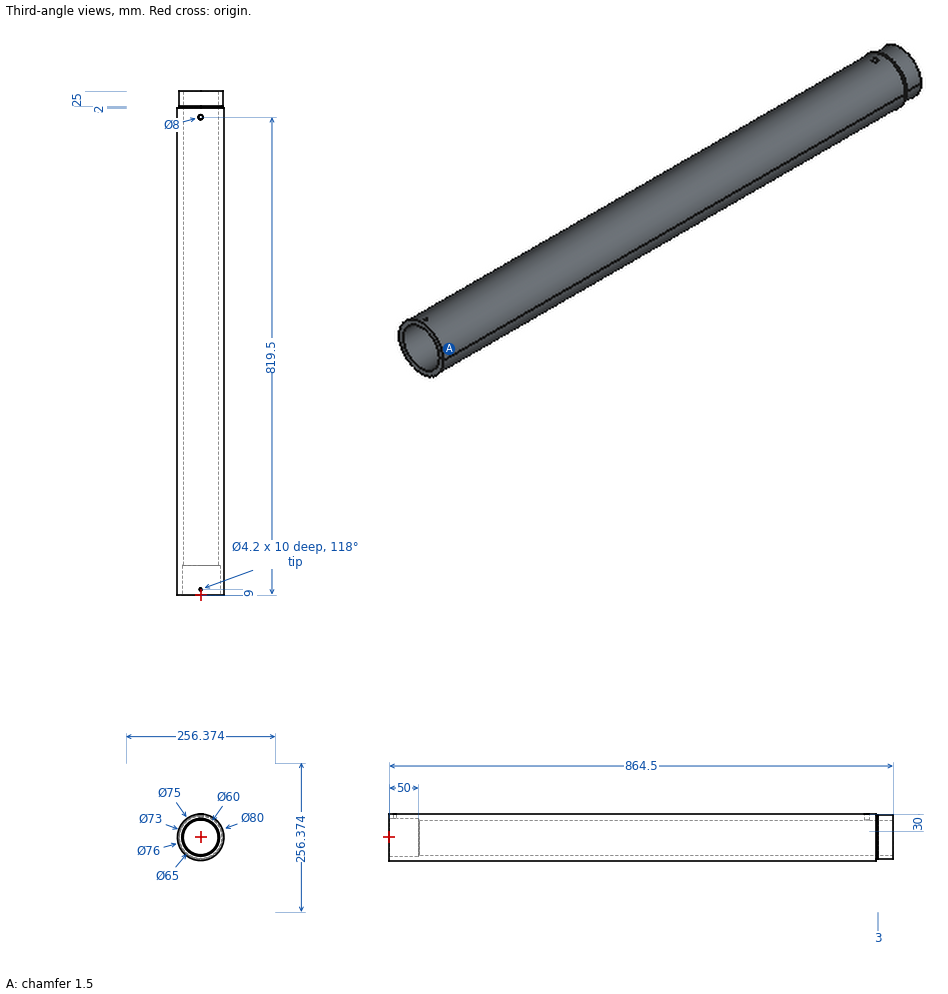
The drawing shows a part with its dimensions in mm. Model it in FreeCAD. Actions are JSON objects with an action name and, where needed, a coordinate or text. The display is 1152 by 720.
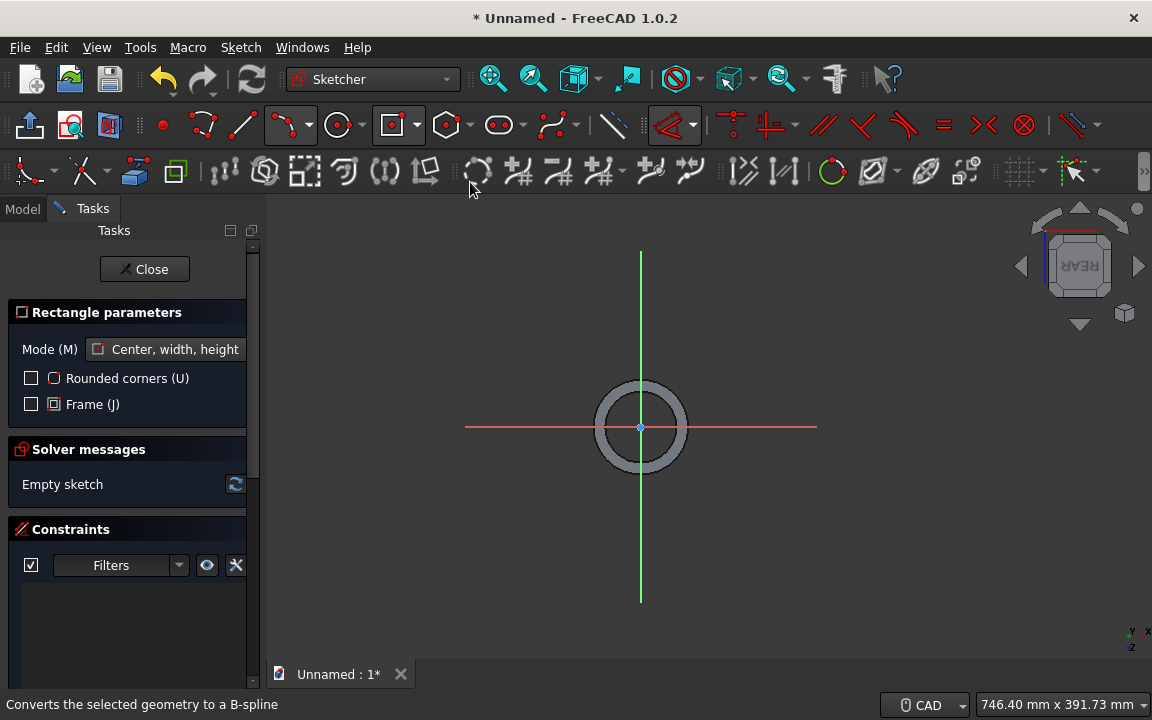
{"action": "left_click", "coordinate": [641, 427]}
{"action": "mouse_move", "coordinate": [793, 275]}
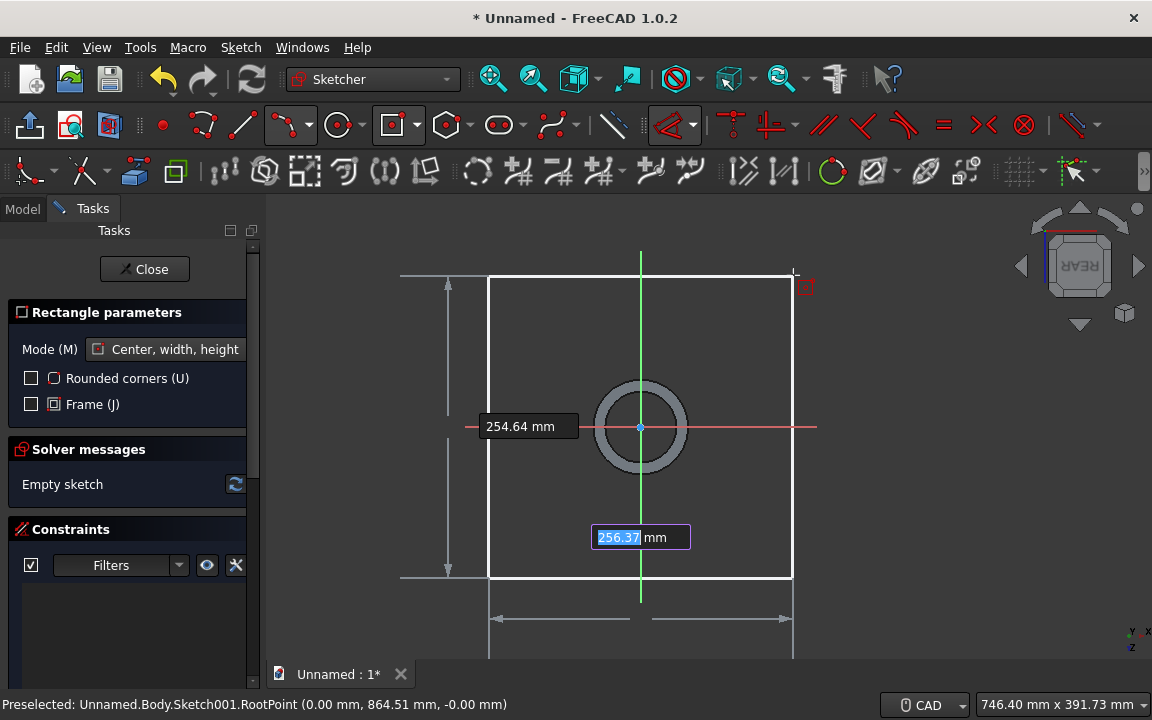
{"action": "type", "text": "256.374"}
{"action": "key", "text": "Tab"}
{"action": "type", "text": "256.374"}
{"action": "key", "text": "Return"}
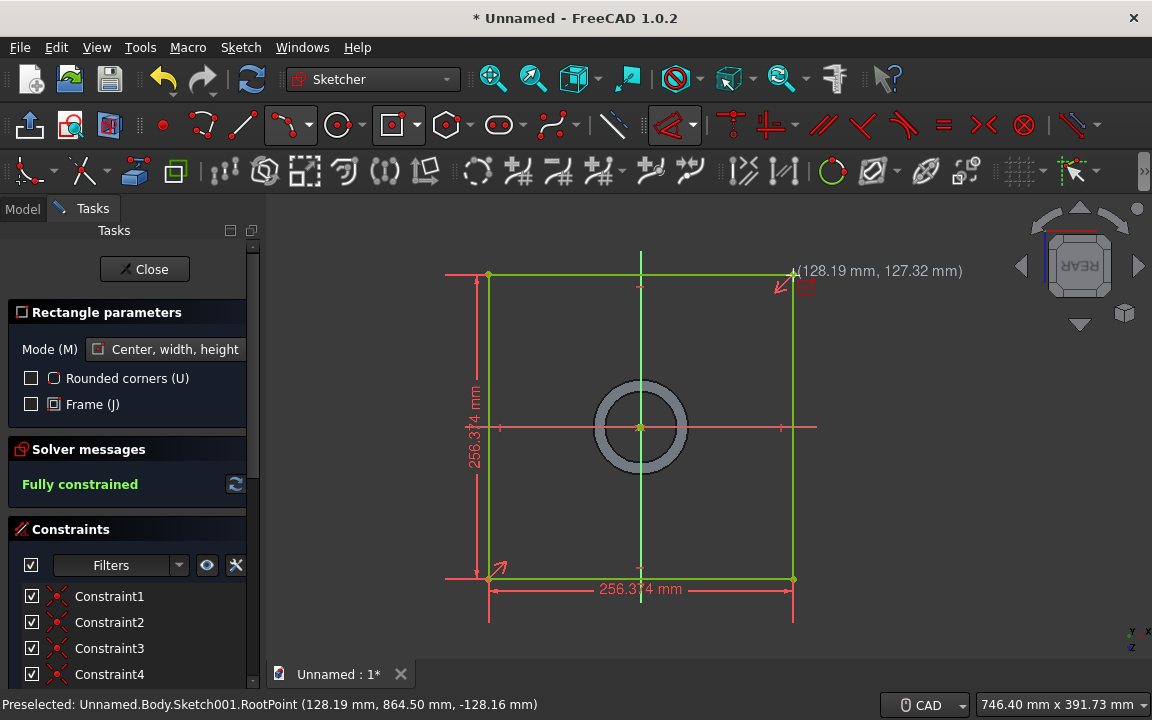
{"action": "left_click", "coordinate": [338, 126]}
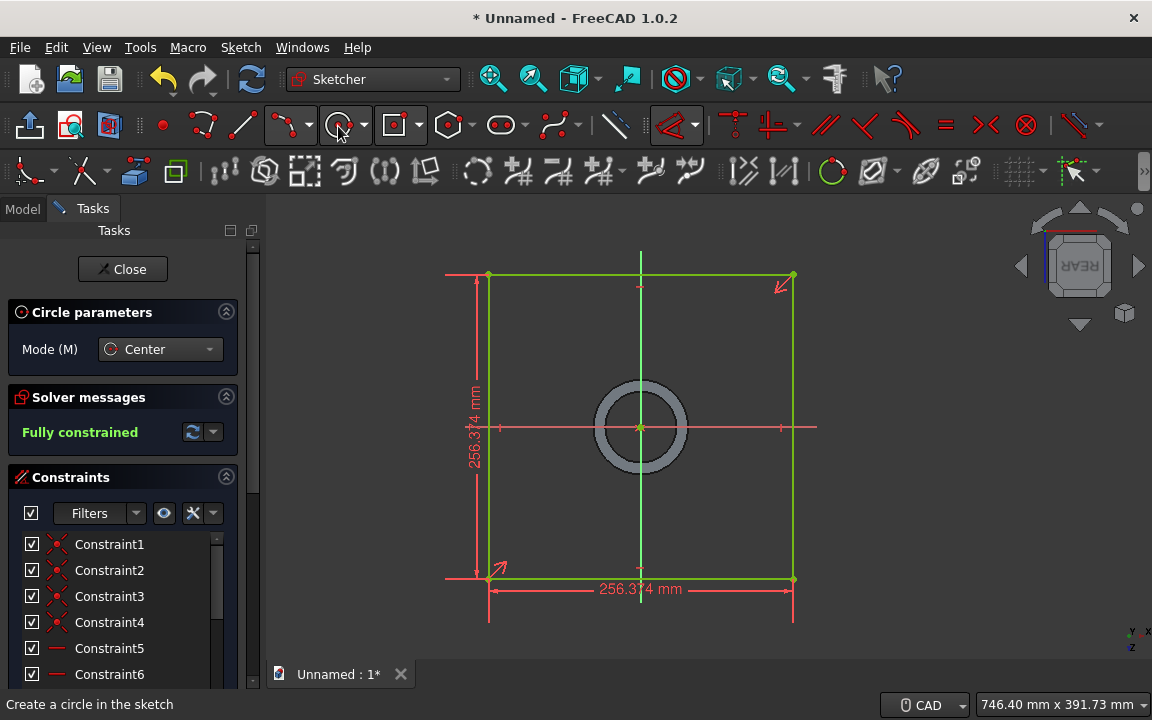
{"action": "left_click", "coordinate": [641, 427]}
{"action": "mouse_move", "coordinate": [672, 396]}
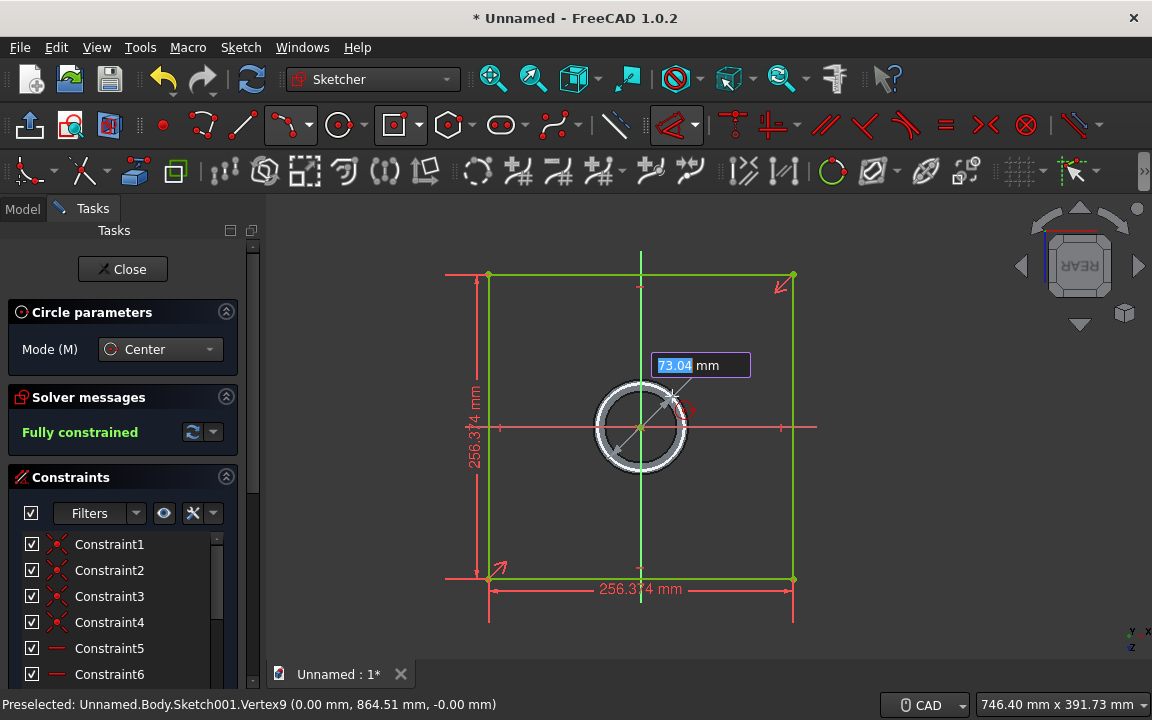
{"action": "type", "text": "75"}
{"action": "key", "text": "Return"}
{"action": "key", "text": "Escape"}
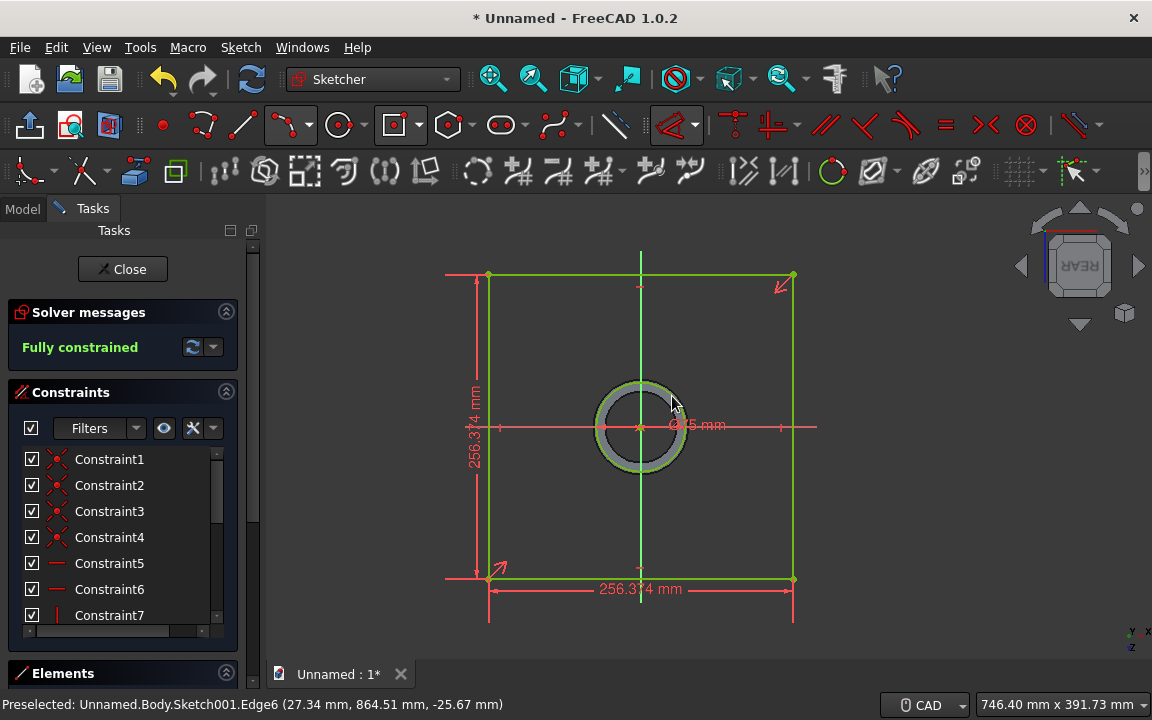
{"action": "left_click", "coordinate": [123, 269]}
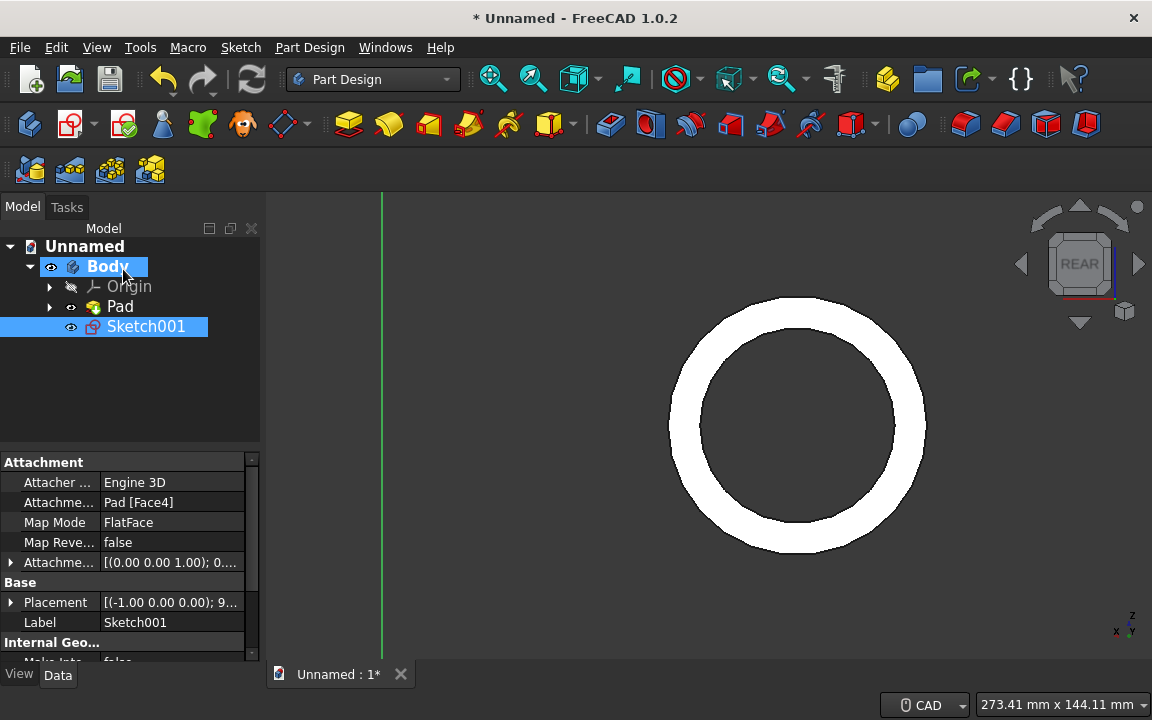
{"action": "left_click", "coordinate": [612, 124]}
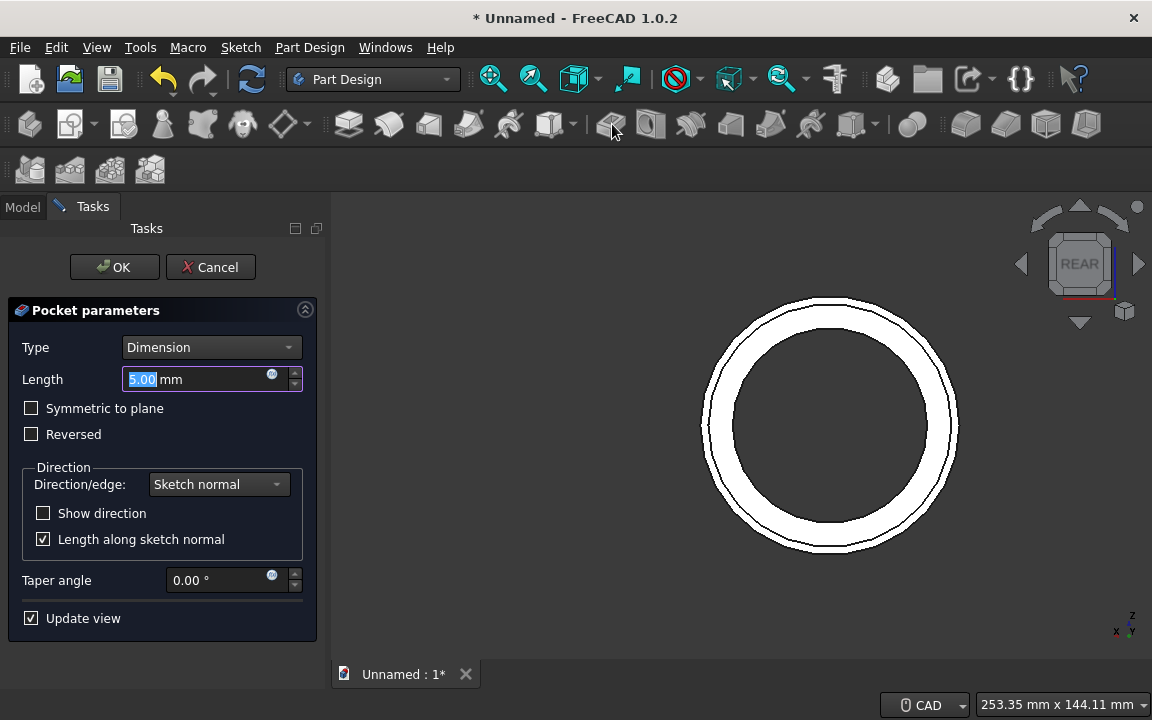
{"action": "type", "text": "25"}
{"action": "key", "text": "Tab"}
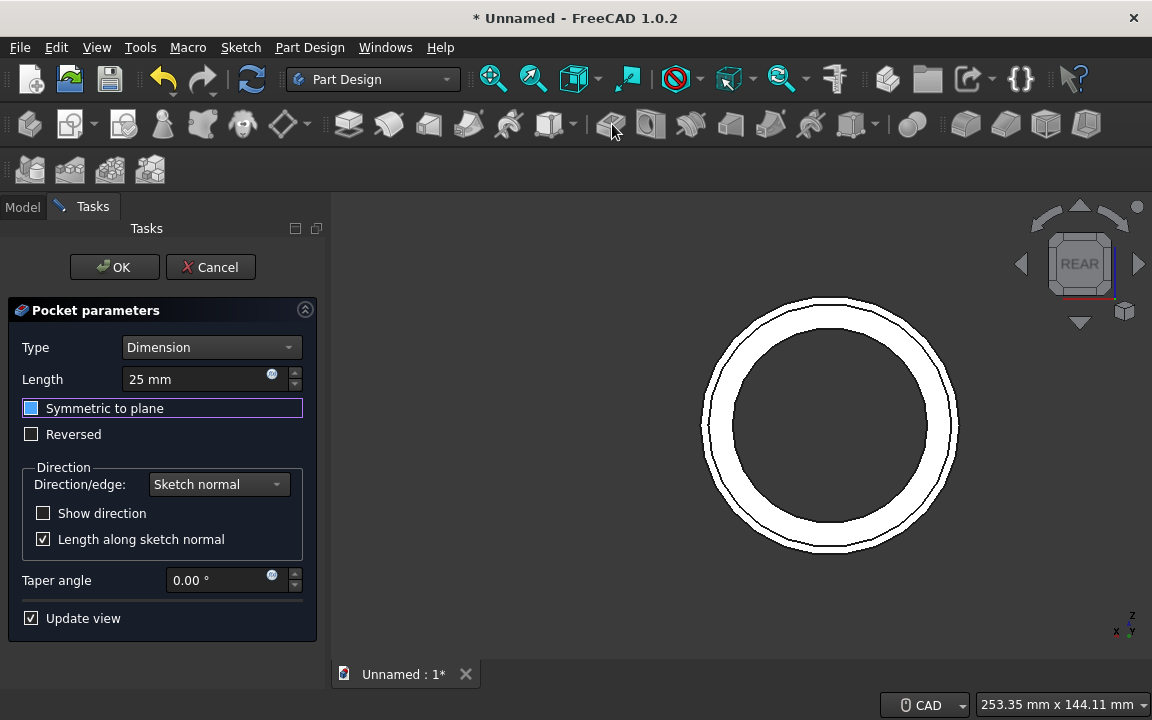
{"action": "left_click", "coordinate": [115, 267]}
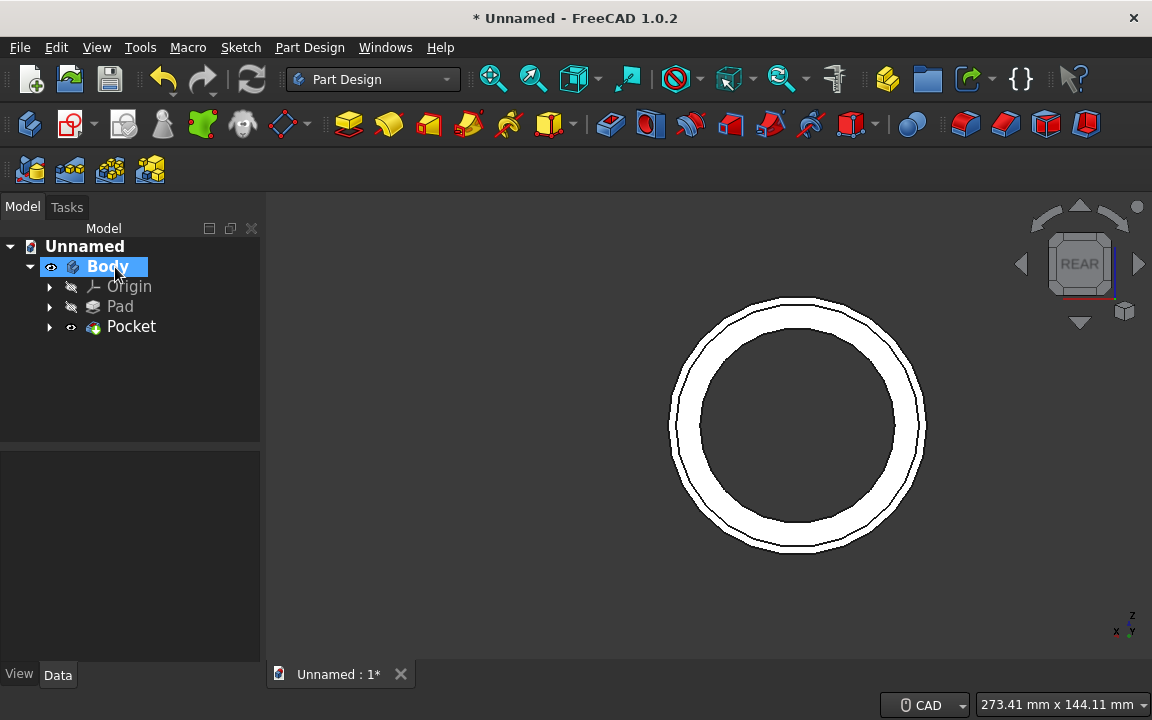
{"action": "scroll", "coordinate": [822, 549], "scroll_direction": "up", "scroll_amount": 8}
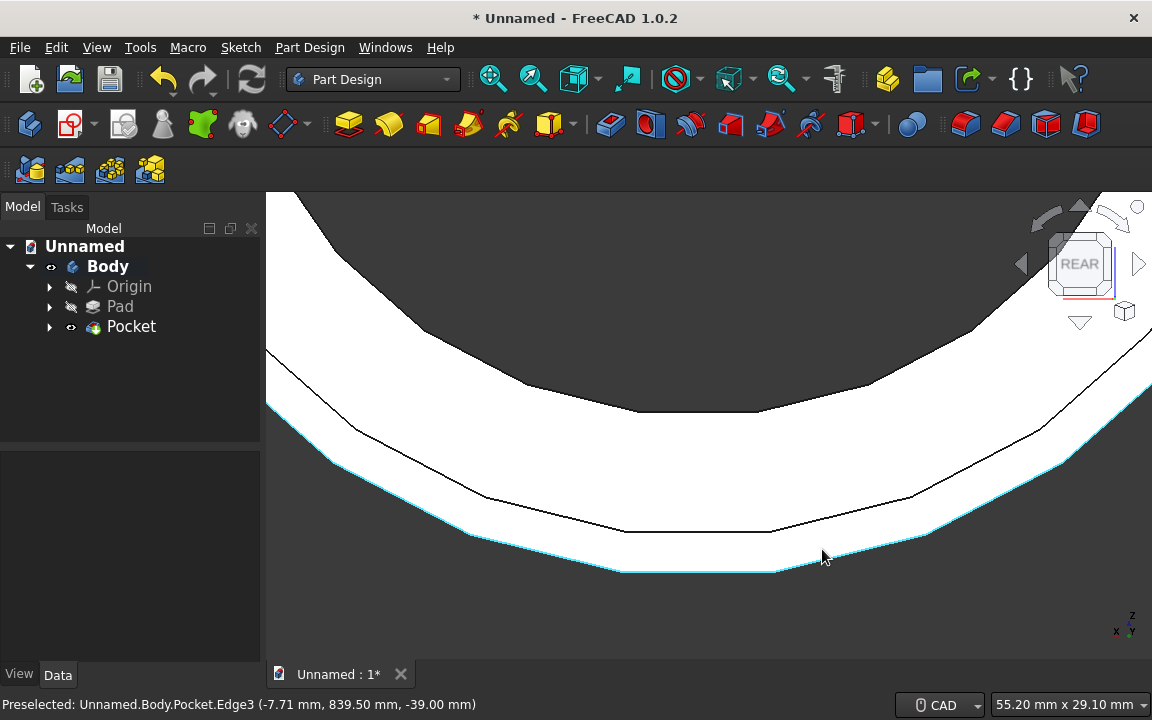
{"action": "left_click", "coordinate": [818, 550]}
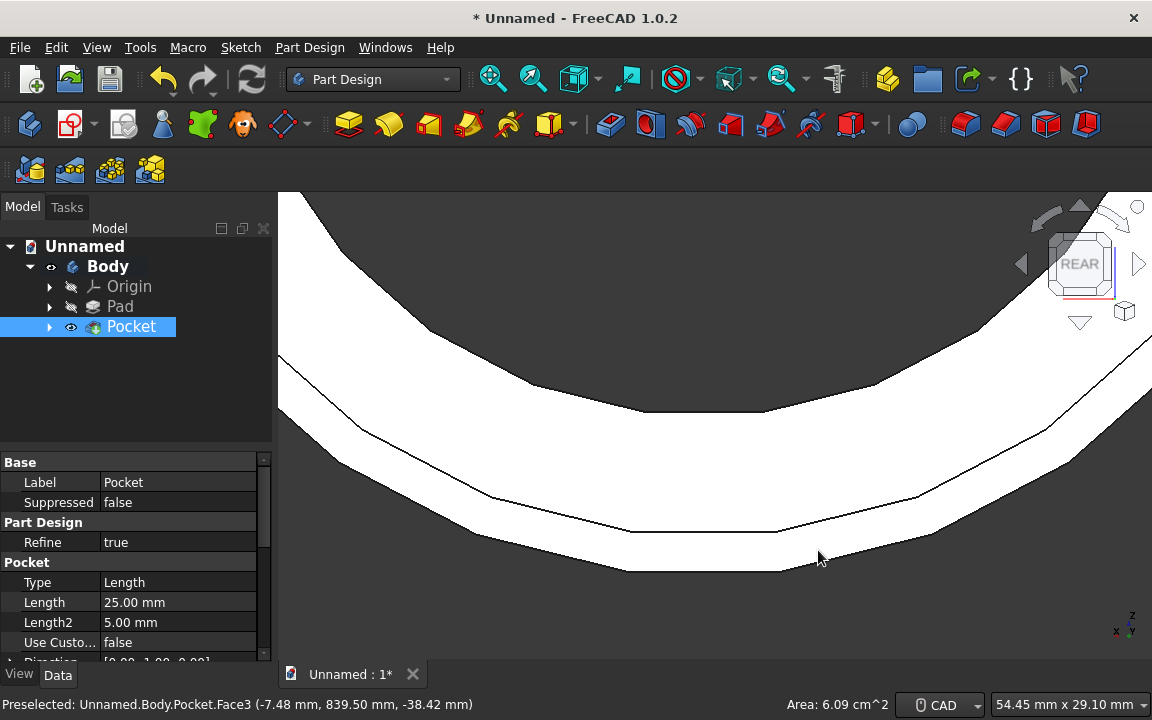
{"action": "left_click", "coordinate": [70, 124]}